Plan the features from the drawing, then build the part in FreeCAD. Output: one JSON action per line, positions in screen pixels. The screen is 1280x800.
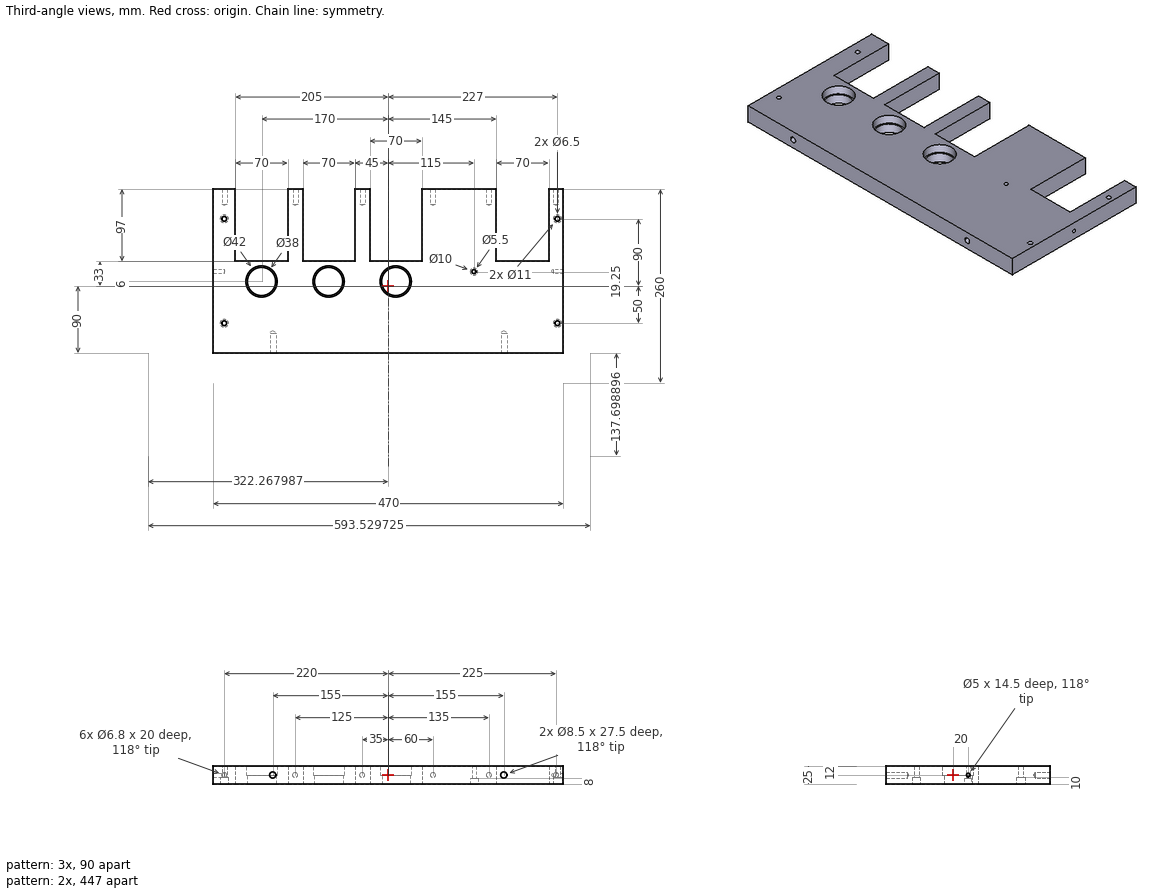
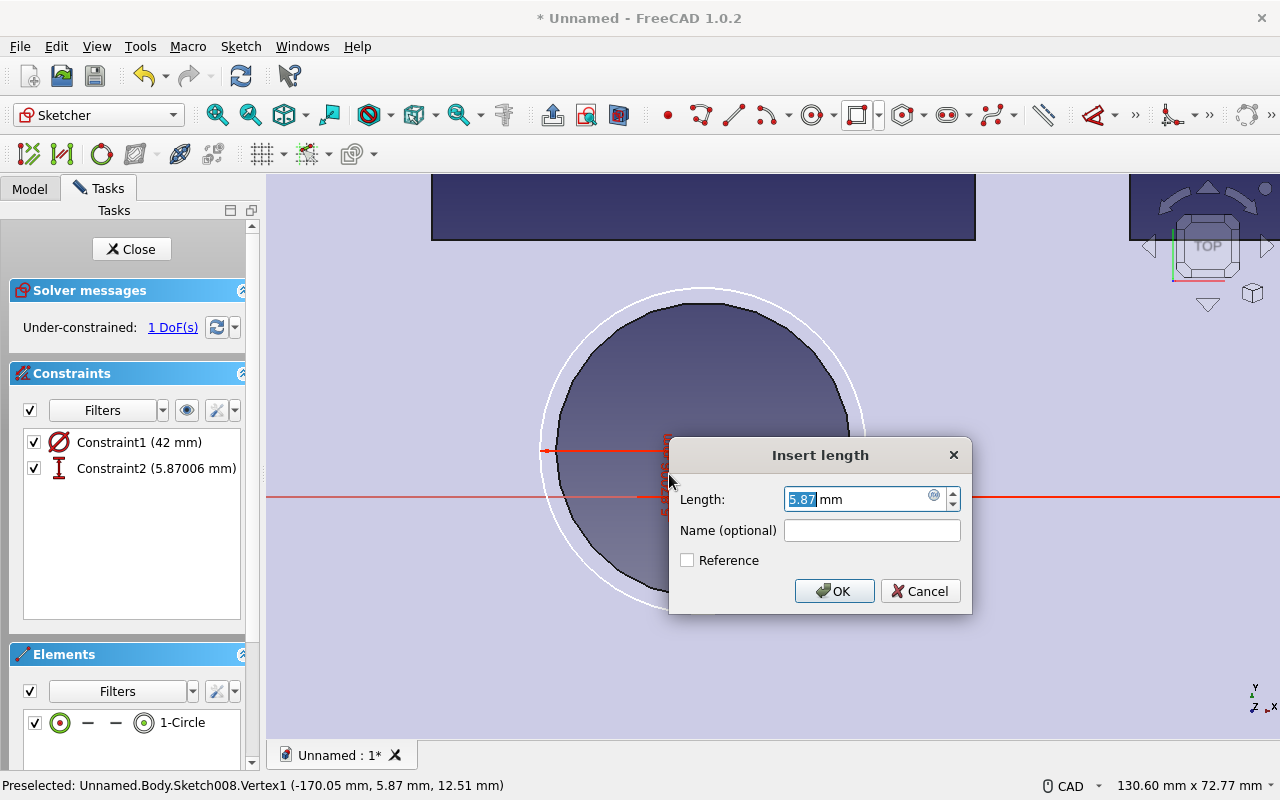
{"action": "type", "text": "6"}
{"action": "key", "text": "Return"}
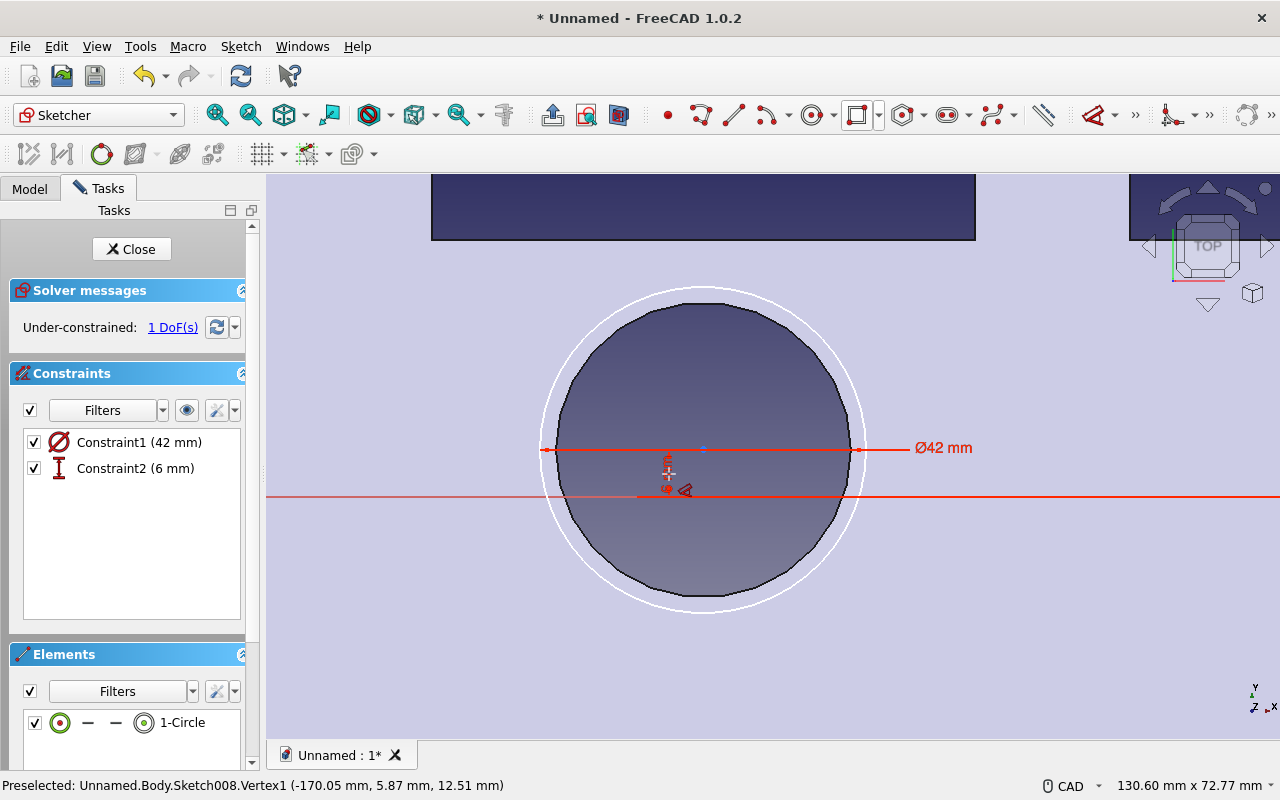
{"action": "left_click", "coordinate": [703, 450]}
{"action": "left_click", "coordinate": [909, 531]}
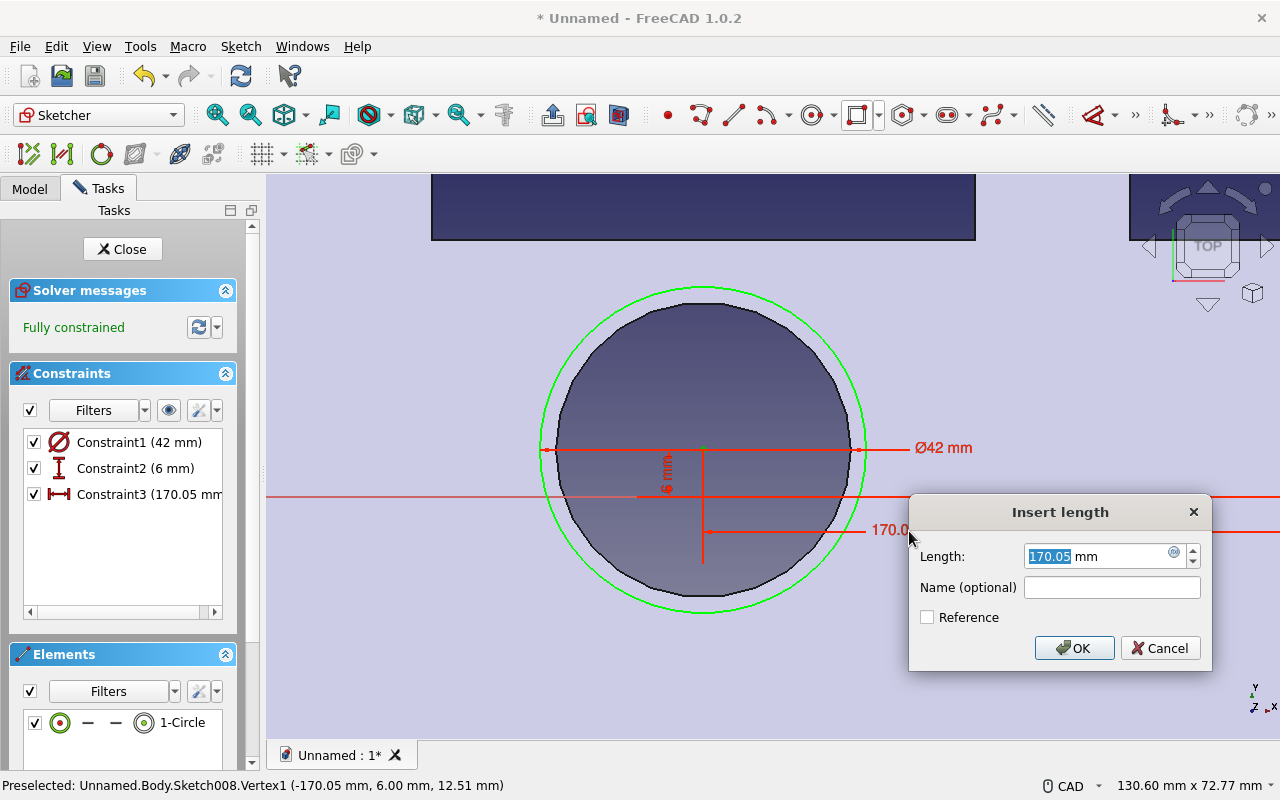
{"action": "type", "text": "170"}
{"action": "key", "text": "Return"}
{"action": "key", "text": "Escape"}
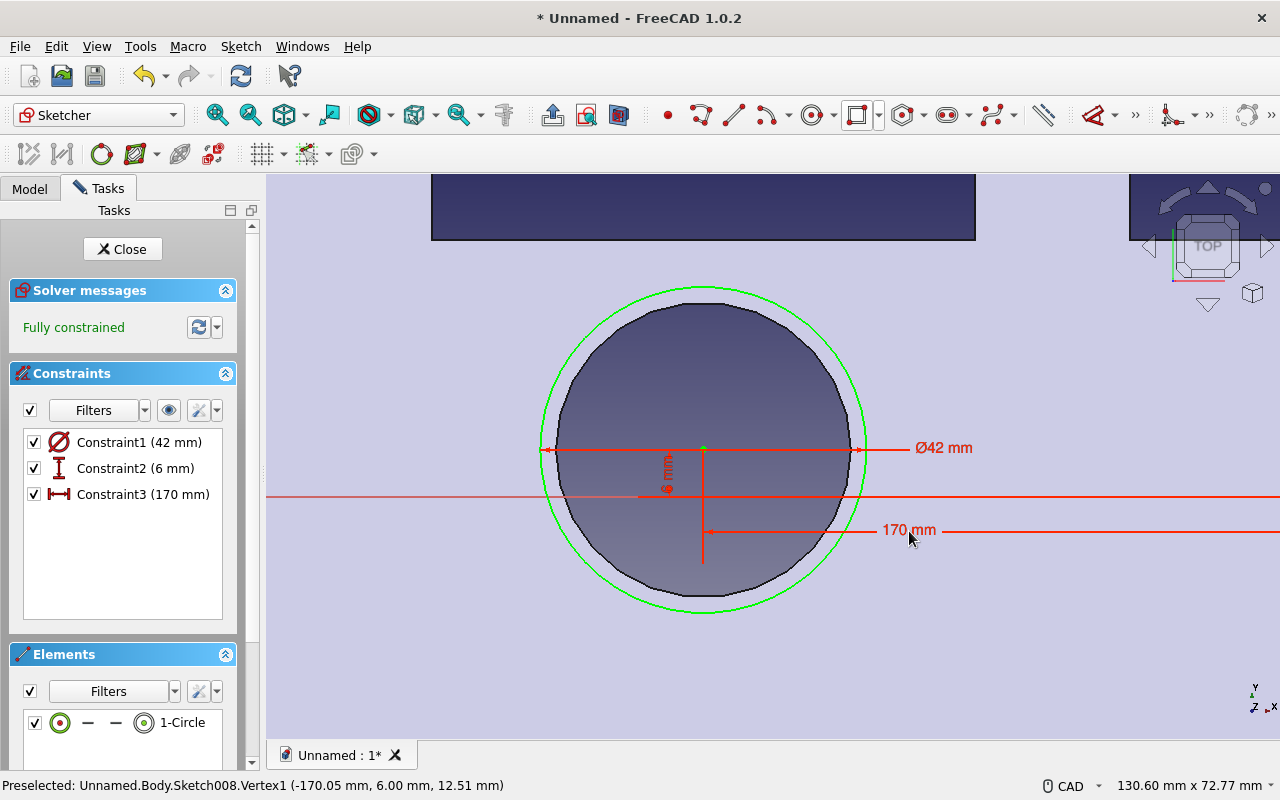
{"action": "left_click", "coordinate": [123, 249]}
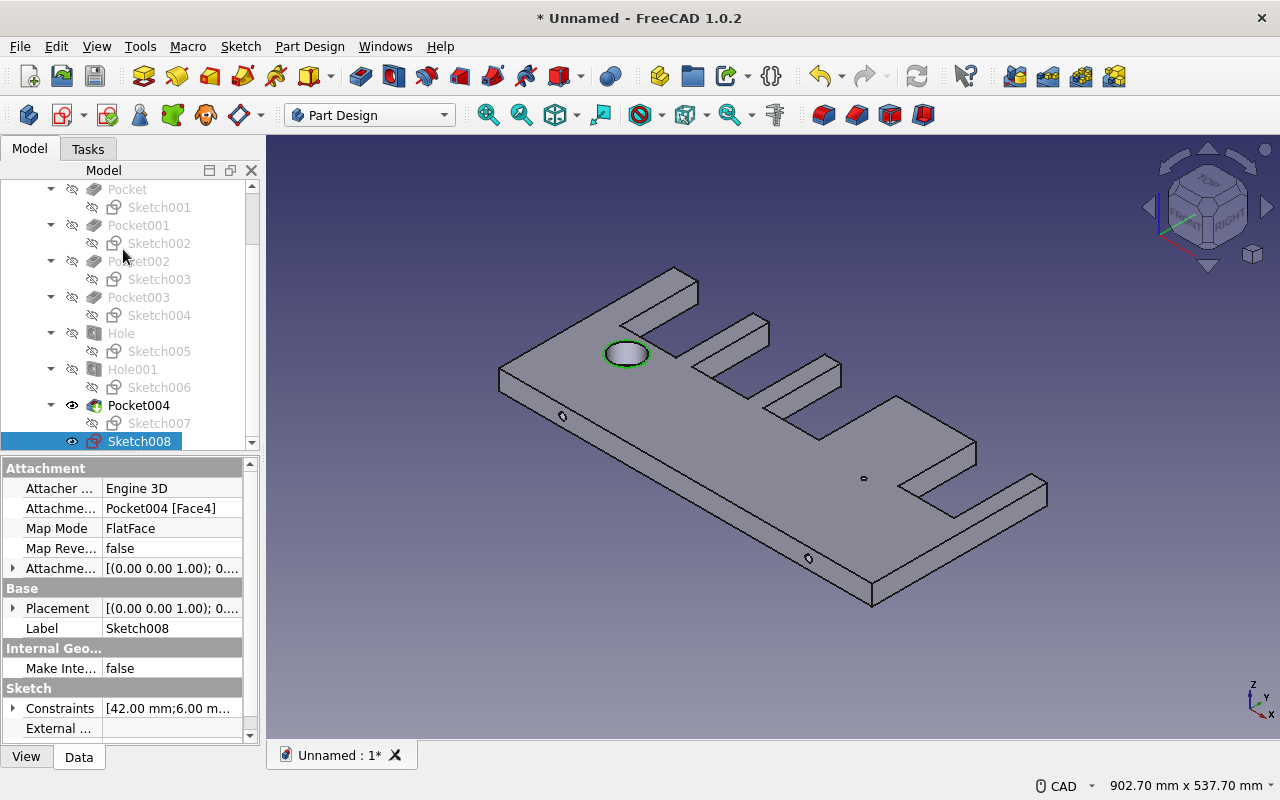
{"action": "left_click", "coordinate": [361, 76]}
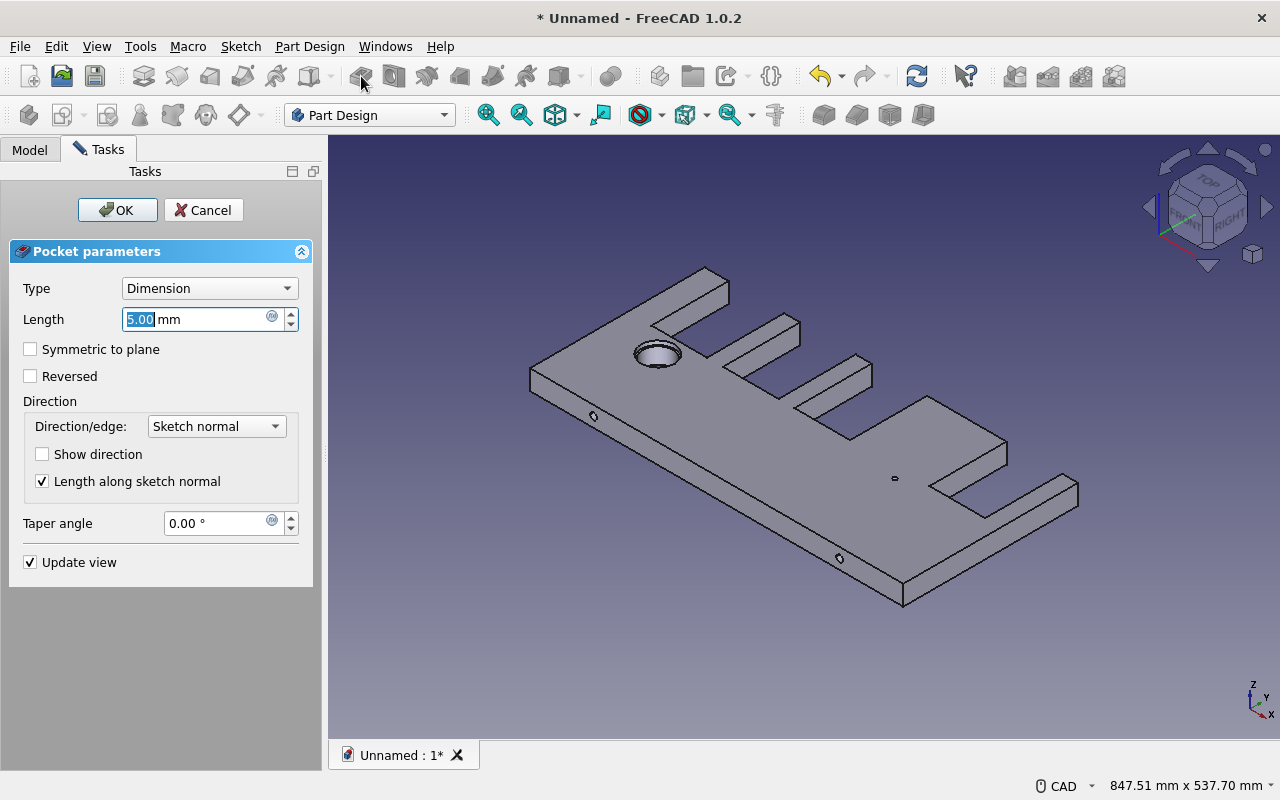
{"action": "type", "text": "12"}
{"action": "key", "text": "Tab"}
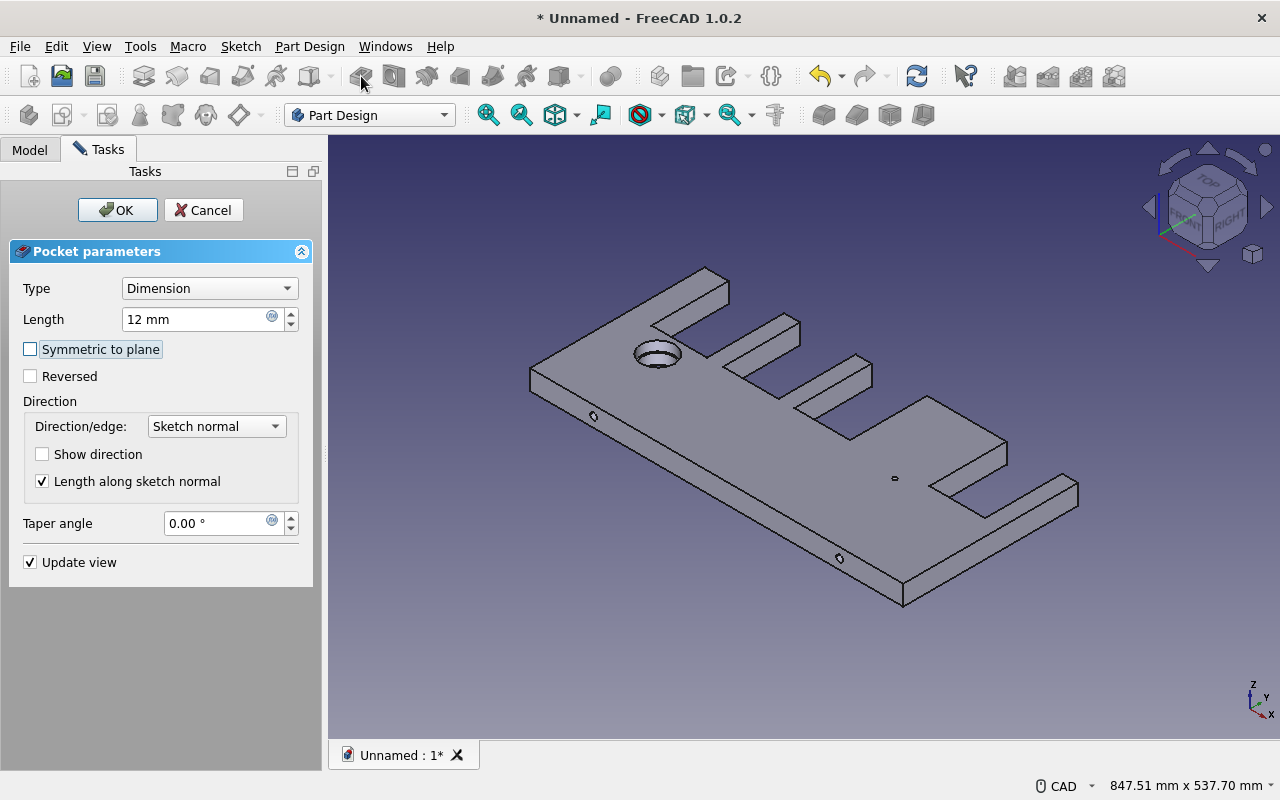
{"action": "left_click", "coordinate": [118, 210]}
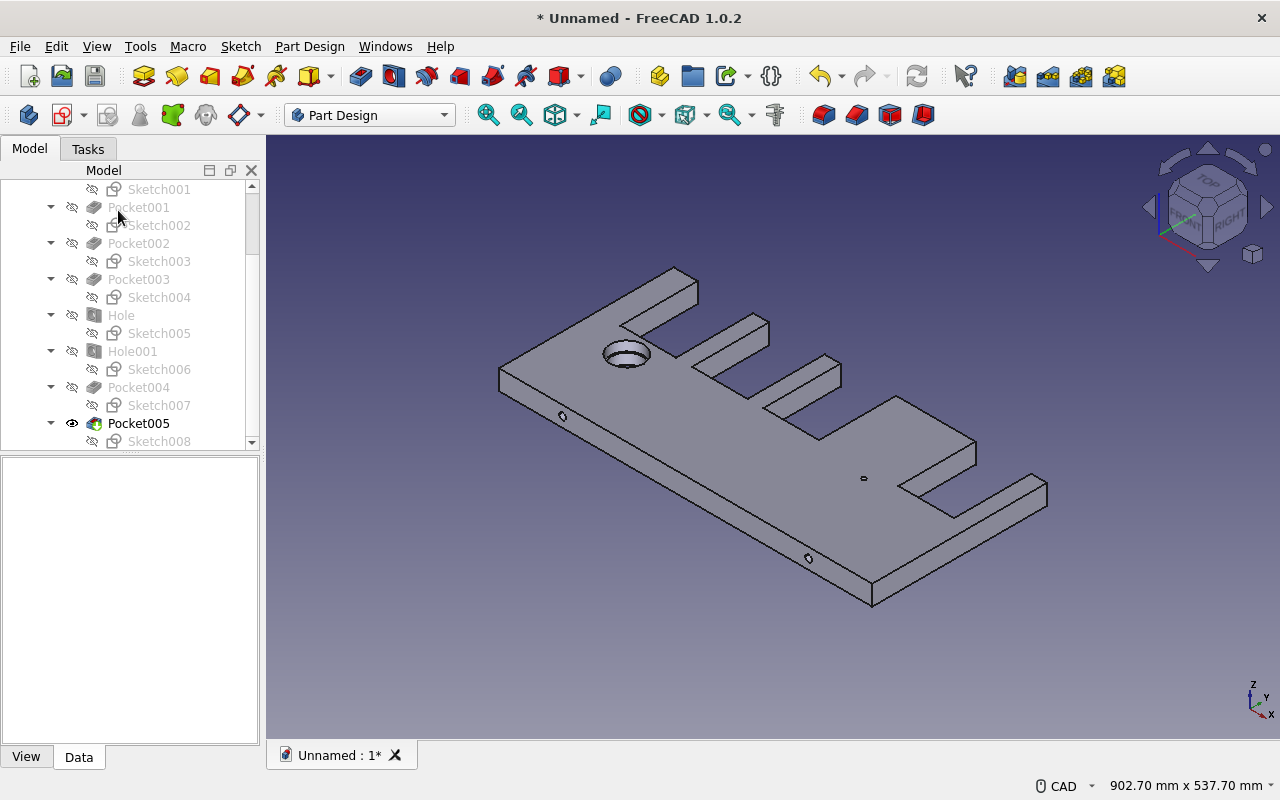
{"action": "left_click", "coordinate": [117, 387]}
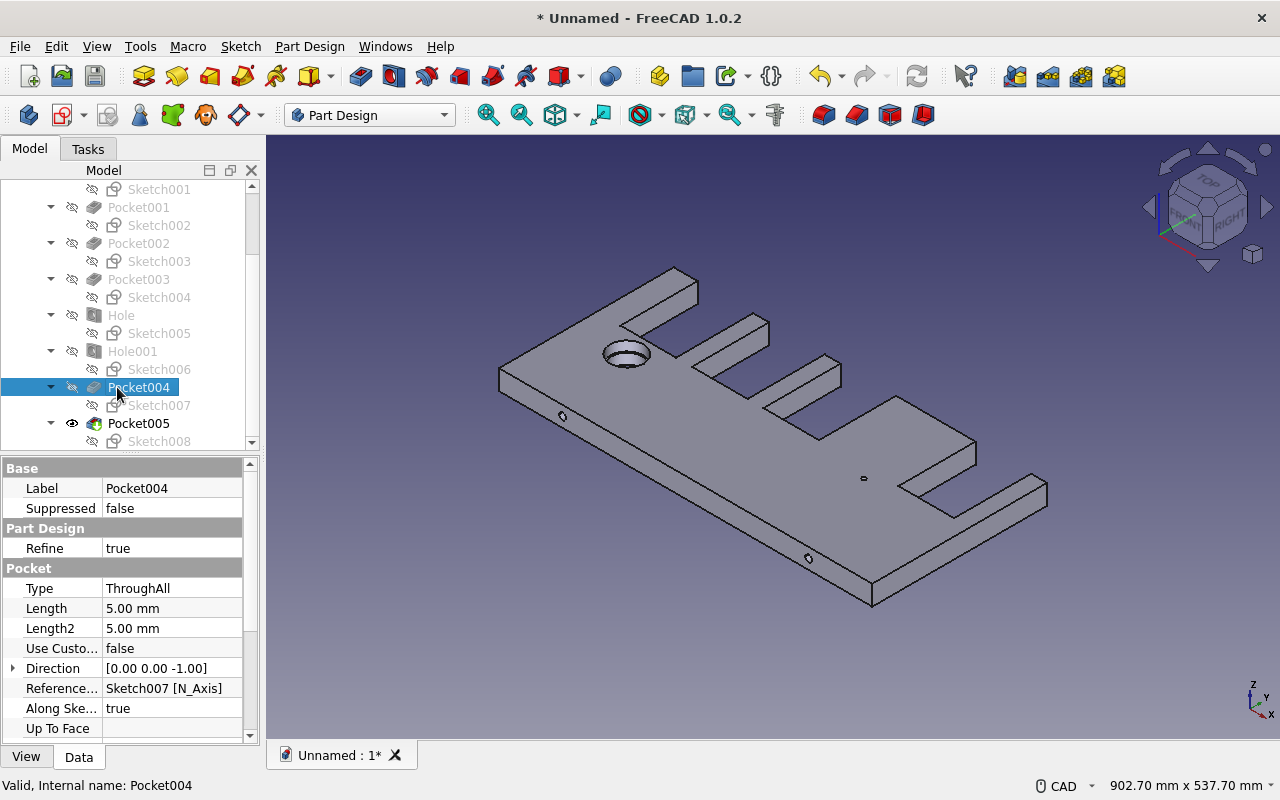
{"action": "left_click", "coordinate": [117, 423], "text": "ctrl"}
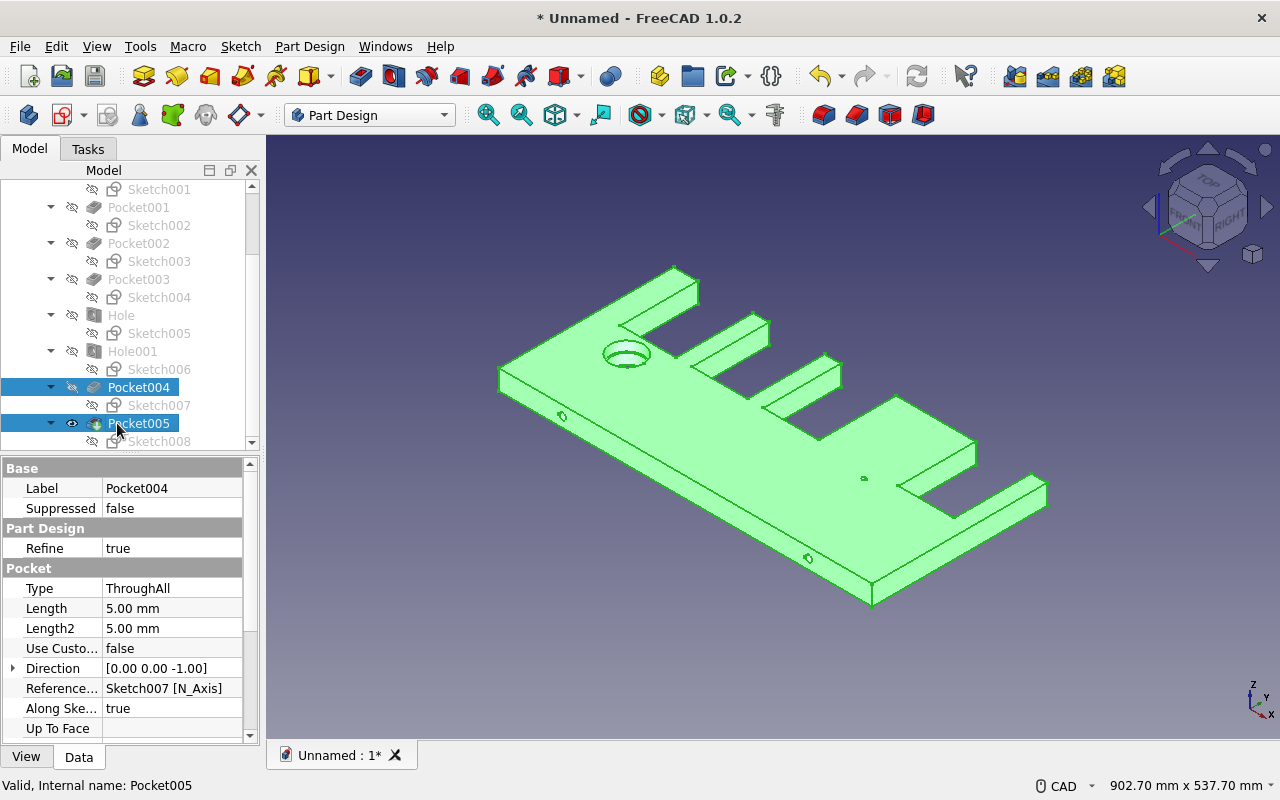
{"action": "left_click", "coordinate": [1048, 76]}